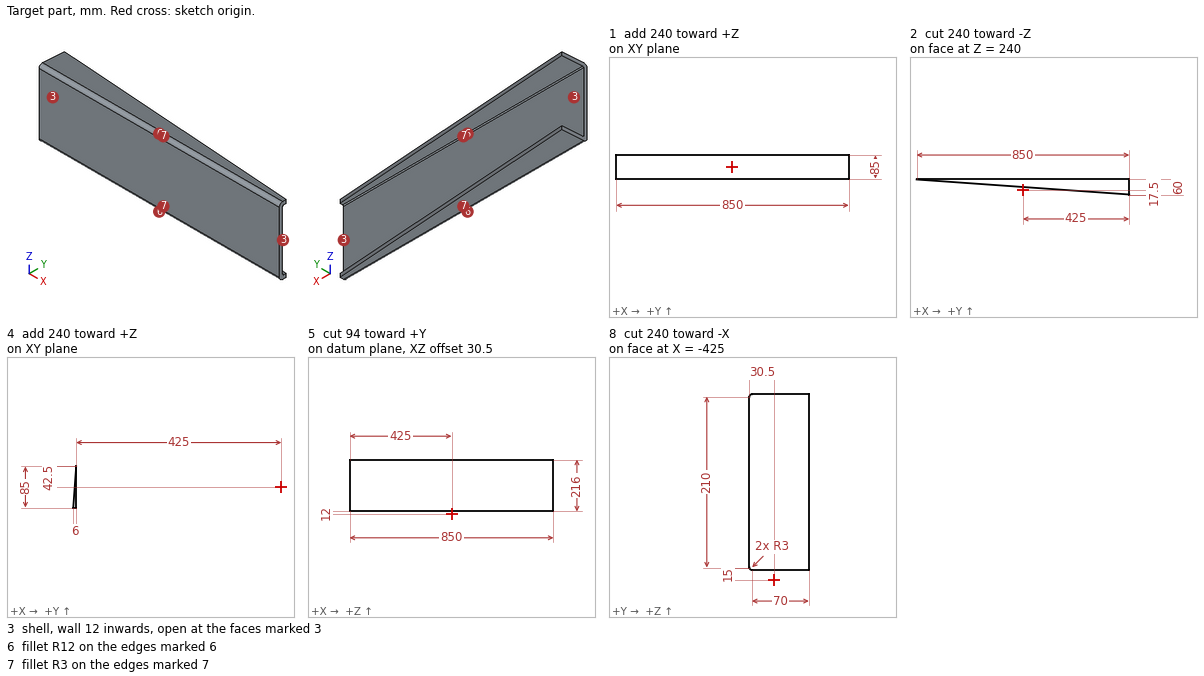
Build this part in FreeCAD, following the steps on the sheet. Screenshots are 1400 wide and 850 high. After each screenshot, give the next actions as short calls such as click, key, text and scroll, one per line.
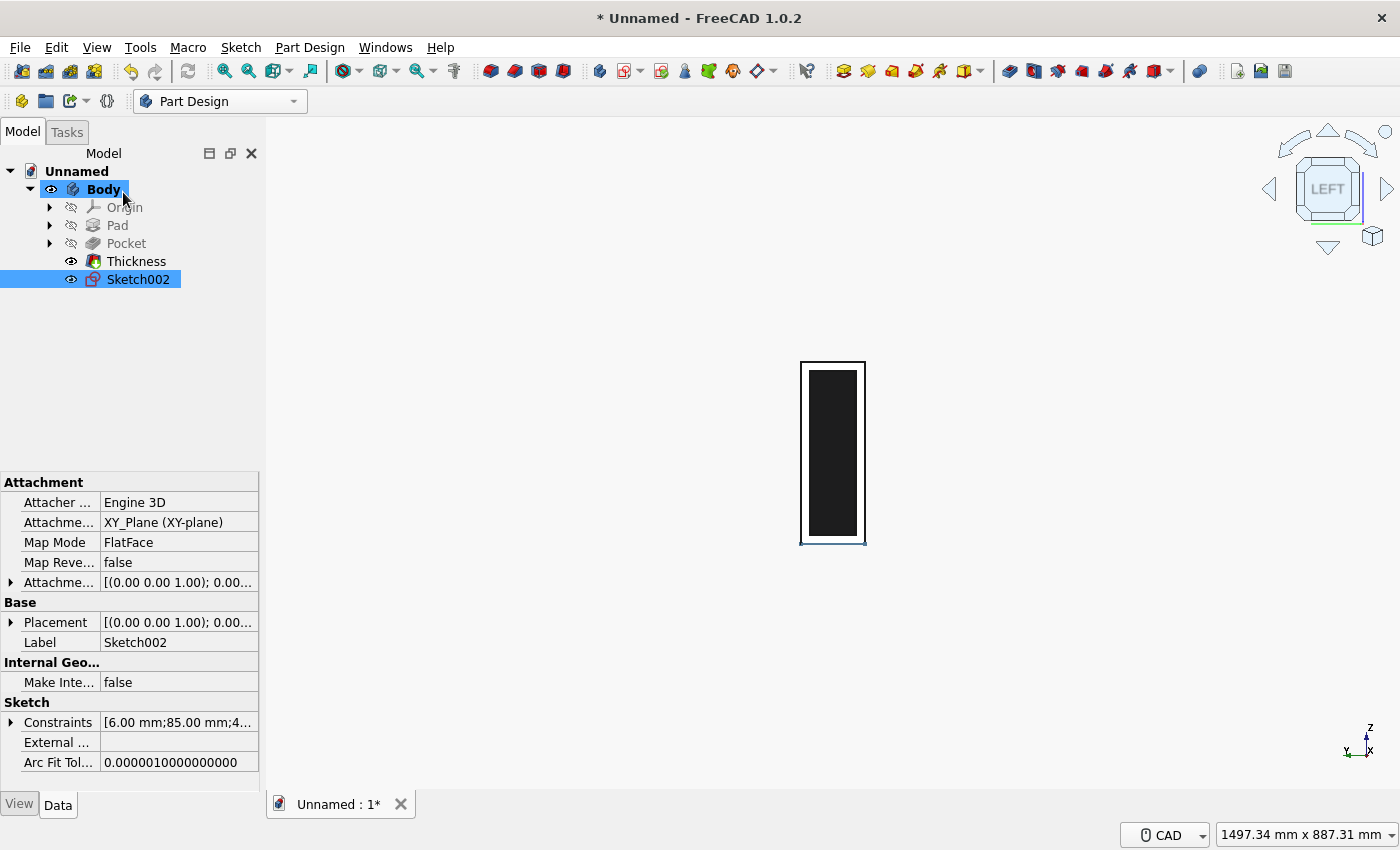
click(844, 72)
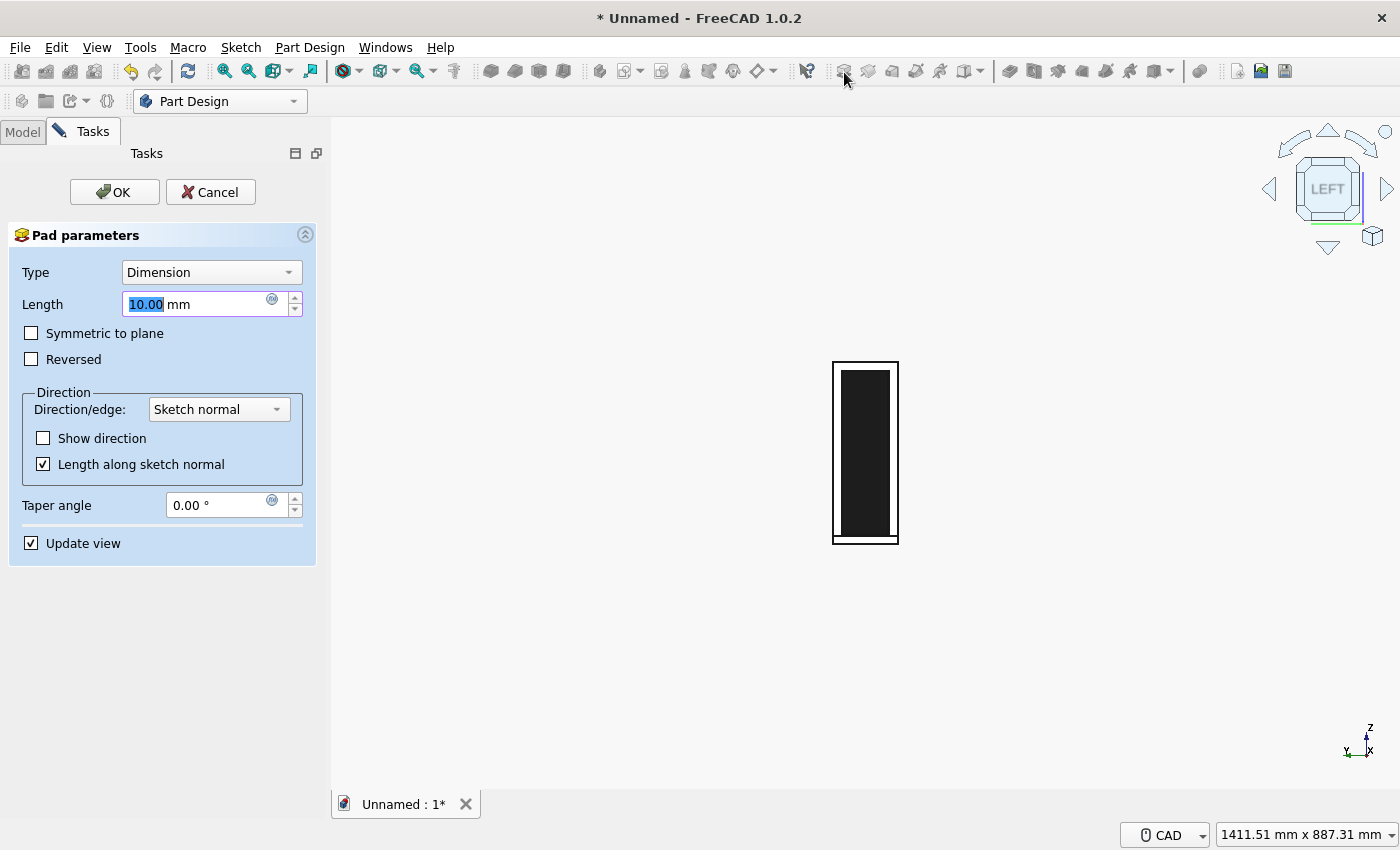
text(240)
key(Tab)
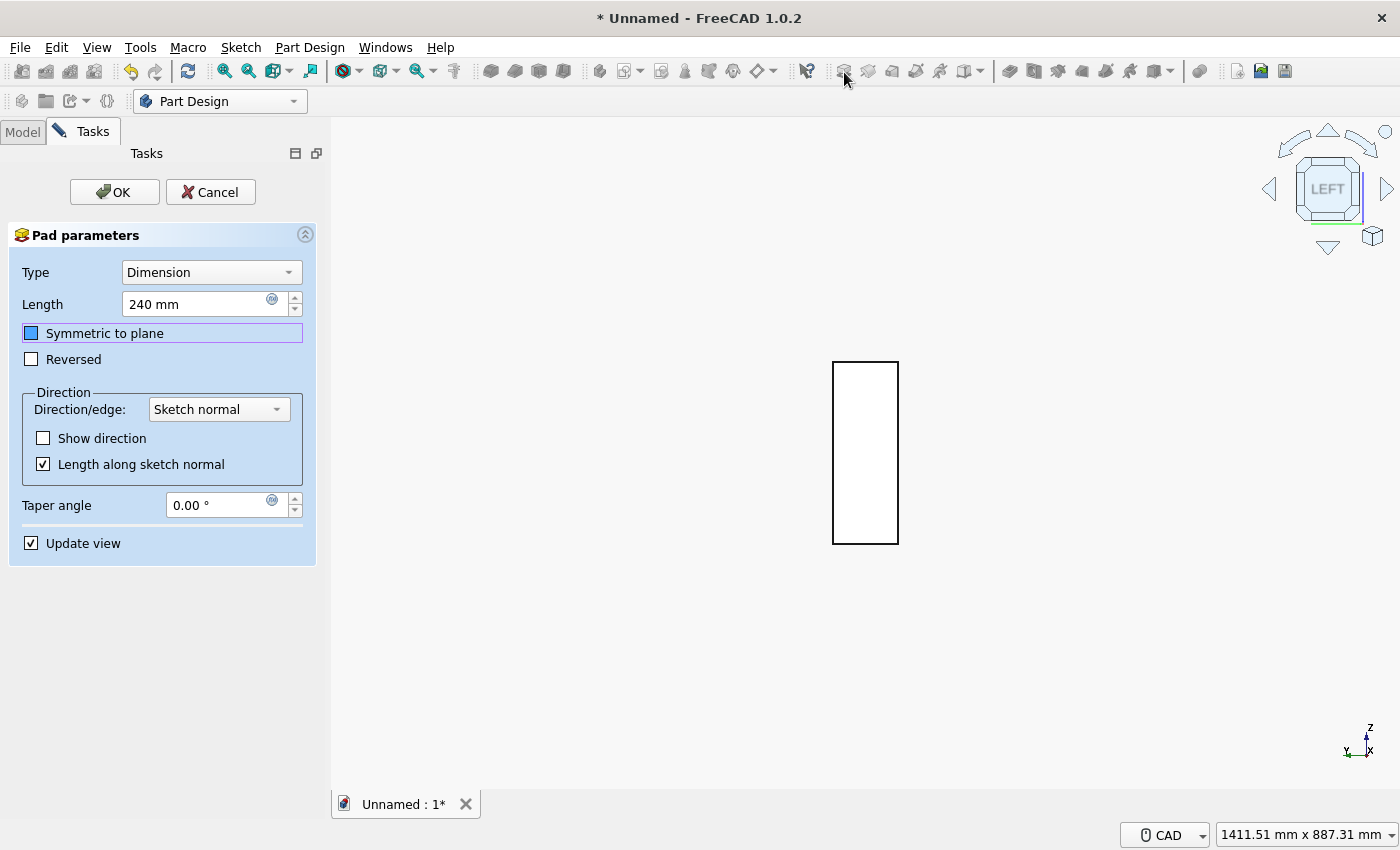
click(115, 192)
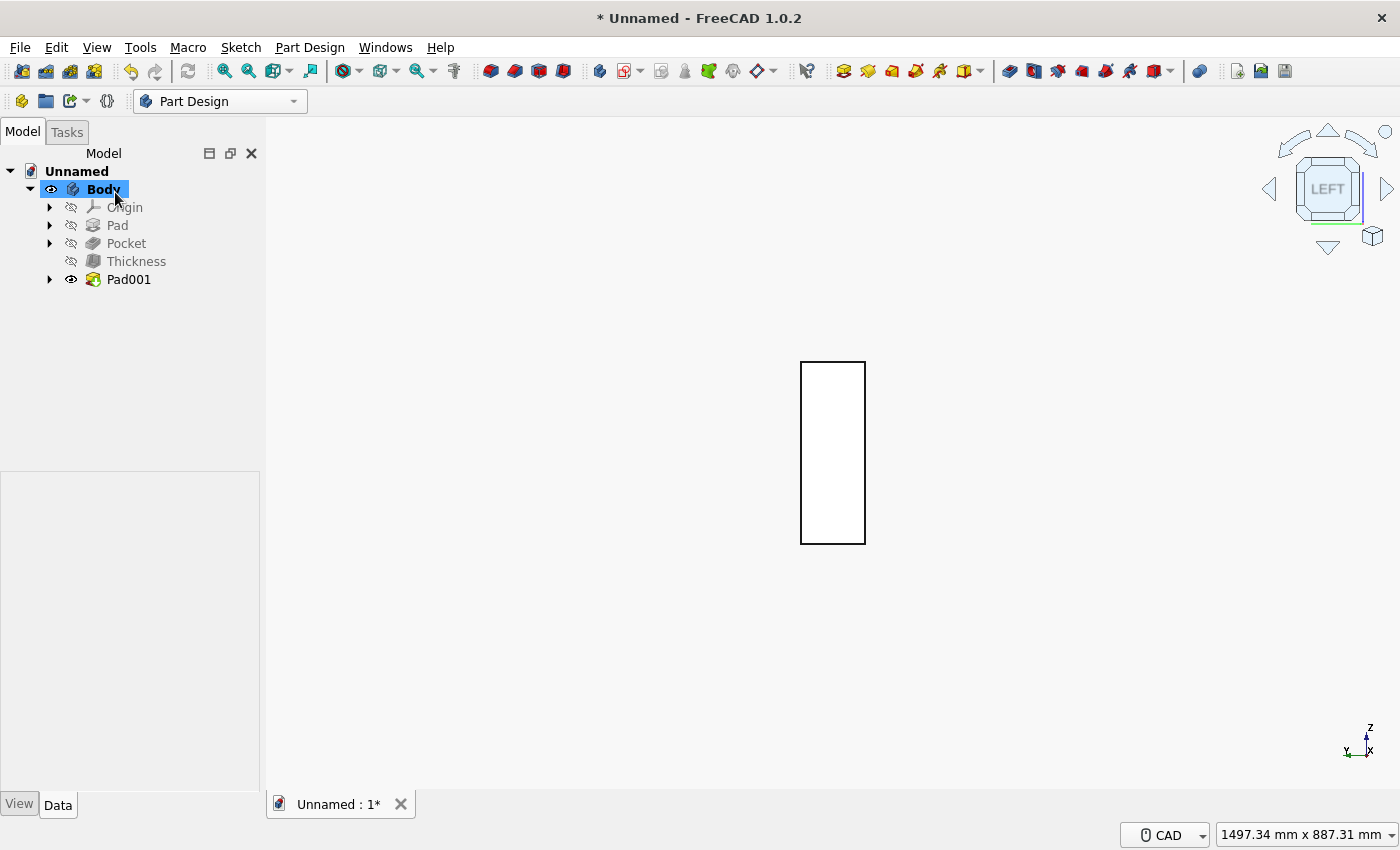
key(v)
key(f)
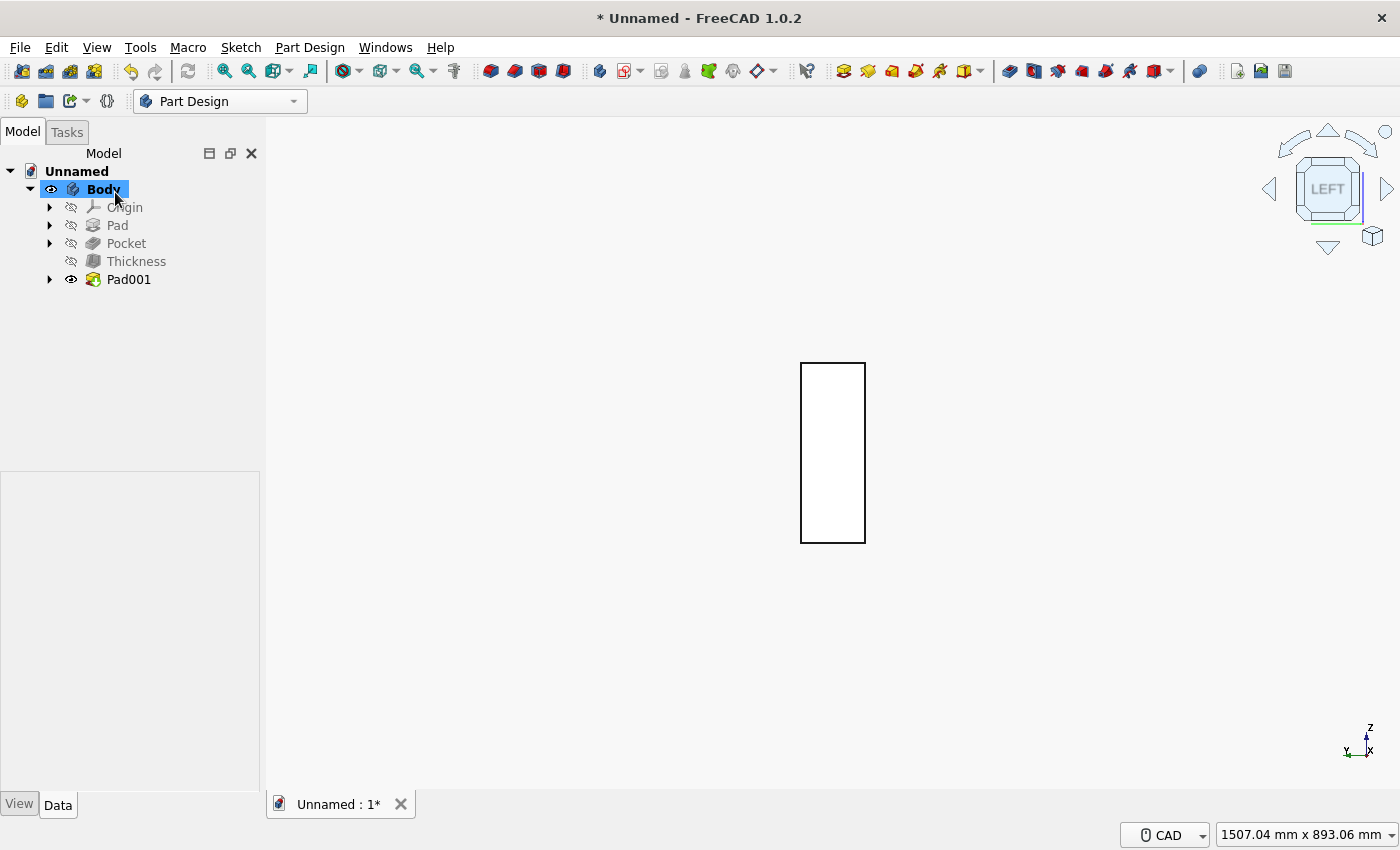
click(50, 207)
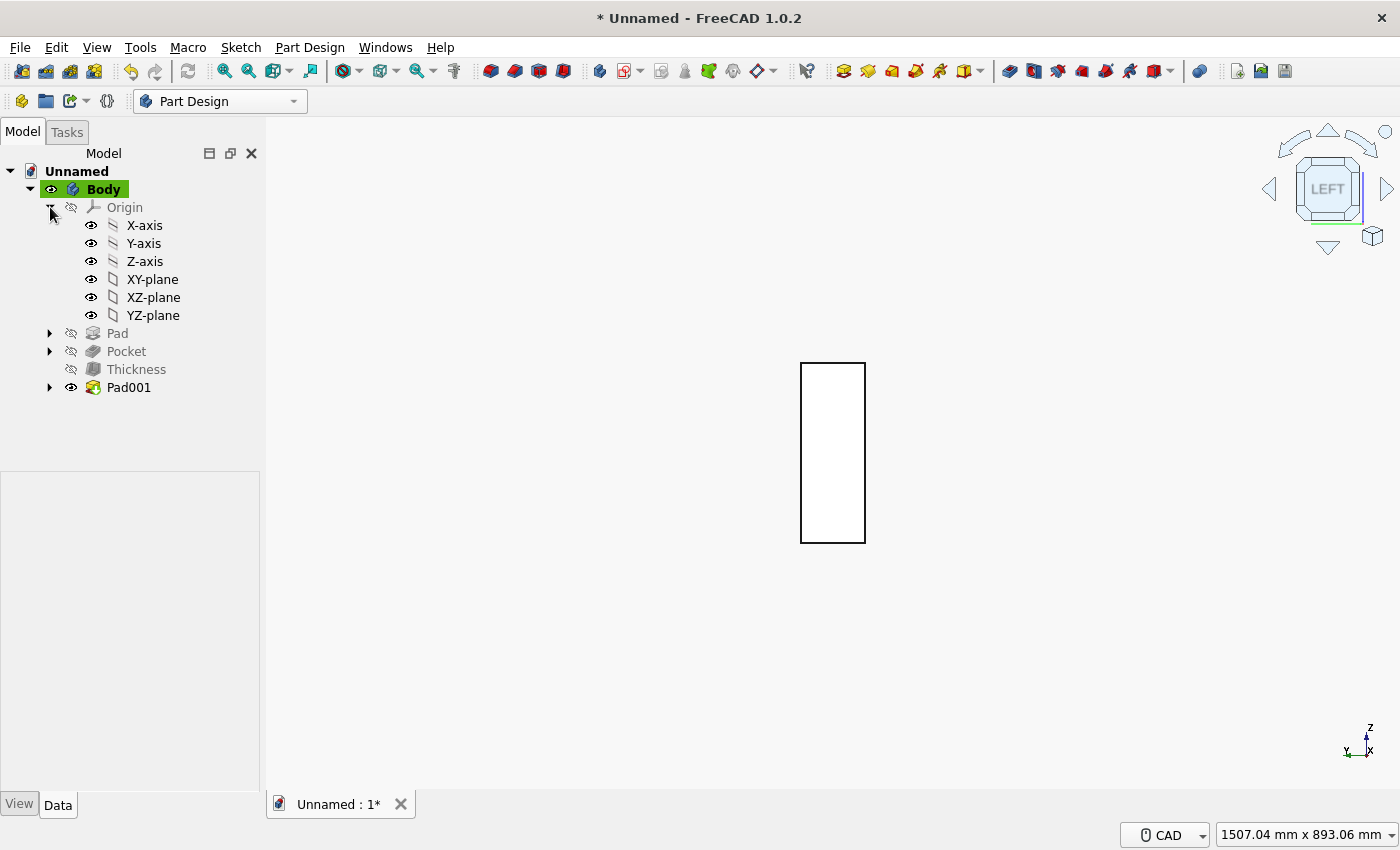
click(136, 297)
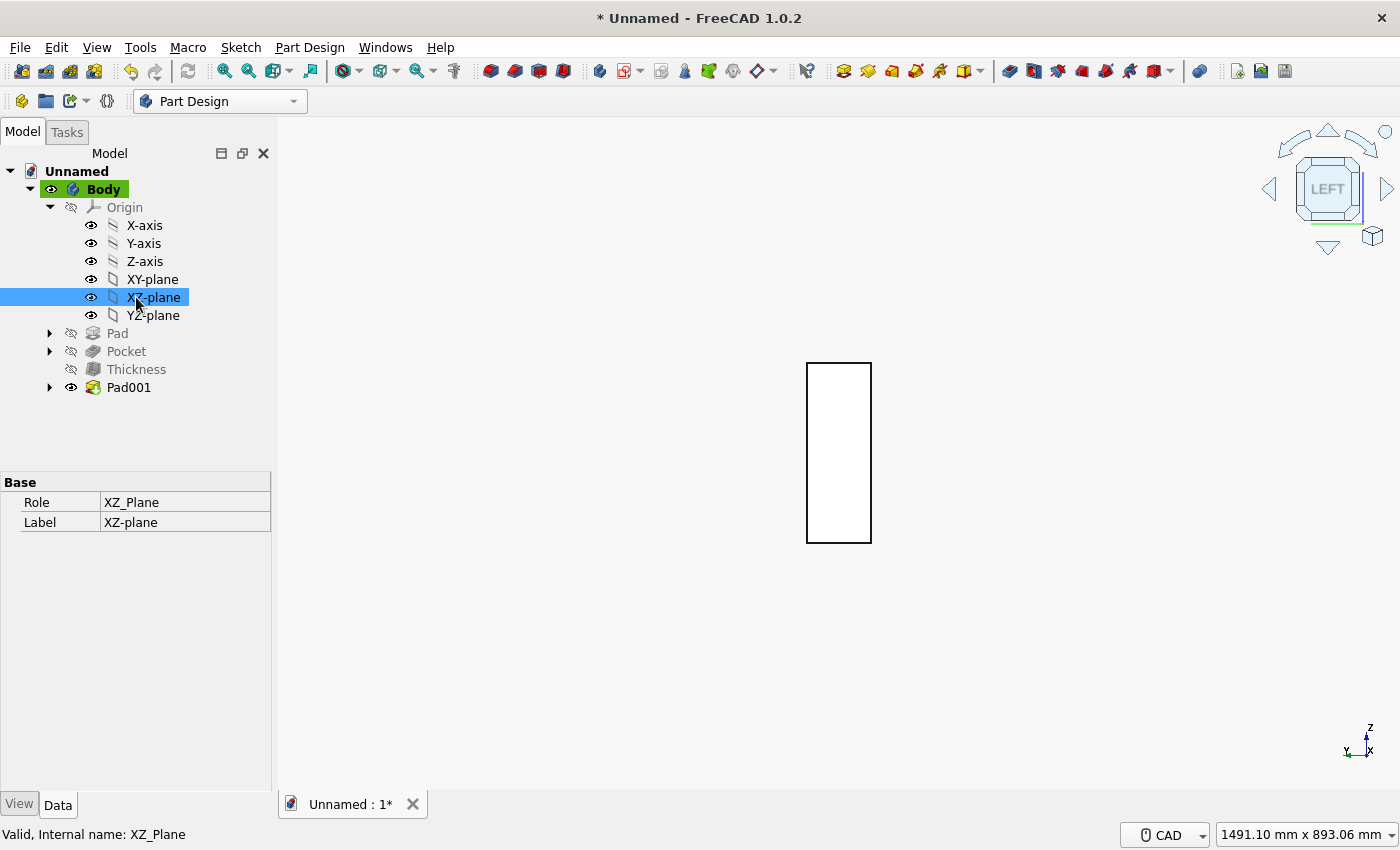
click(758, 72)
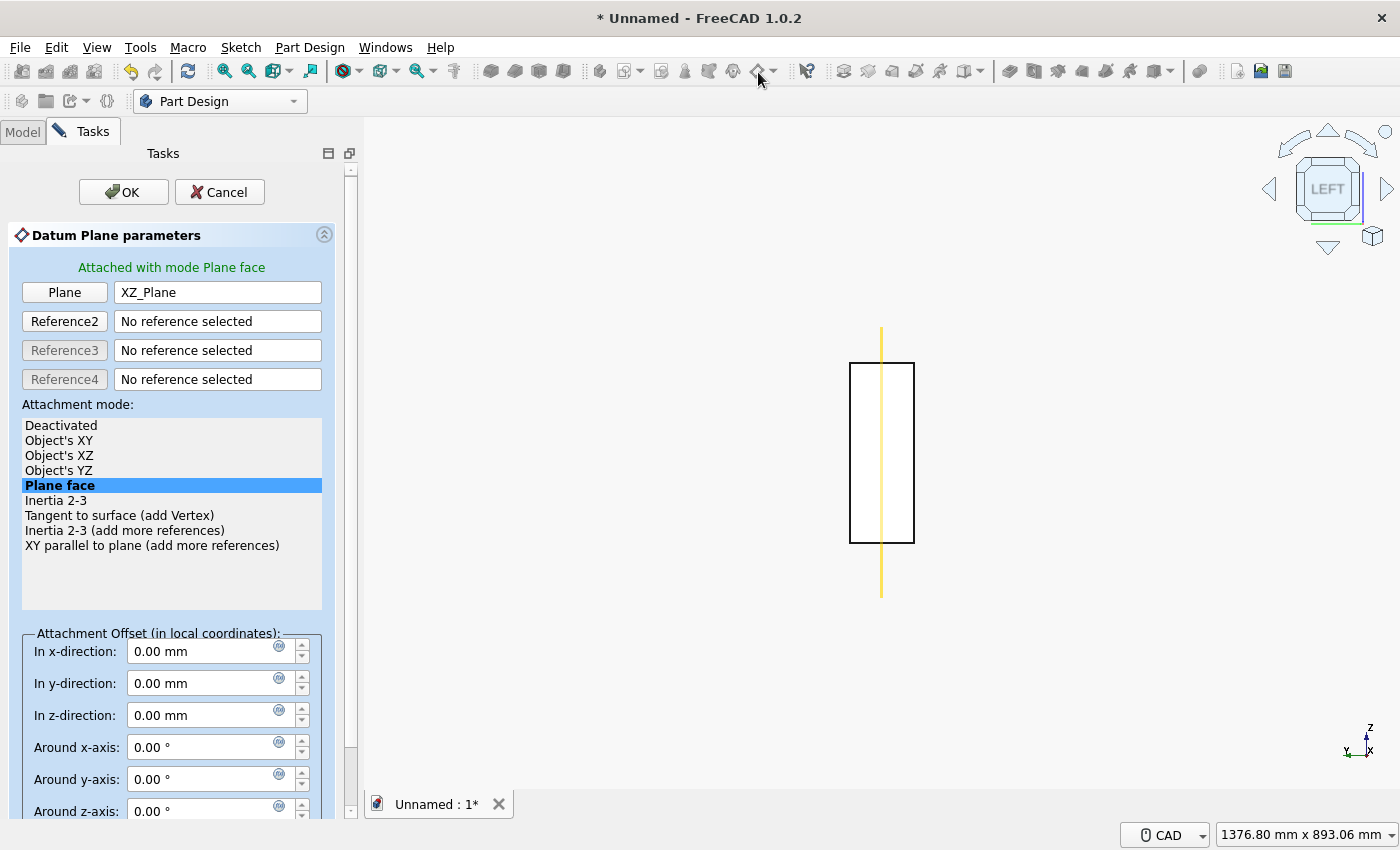
triple_click(210, 715)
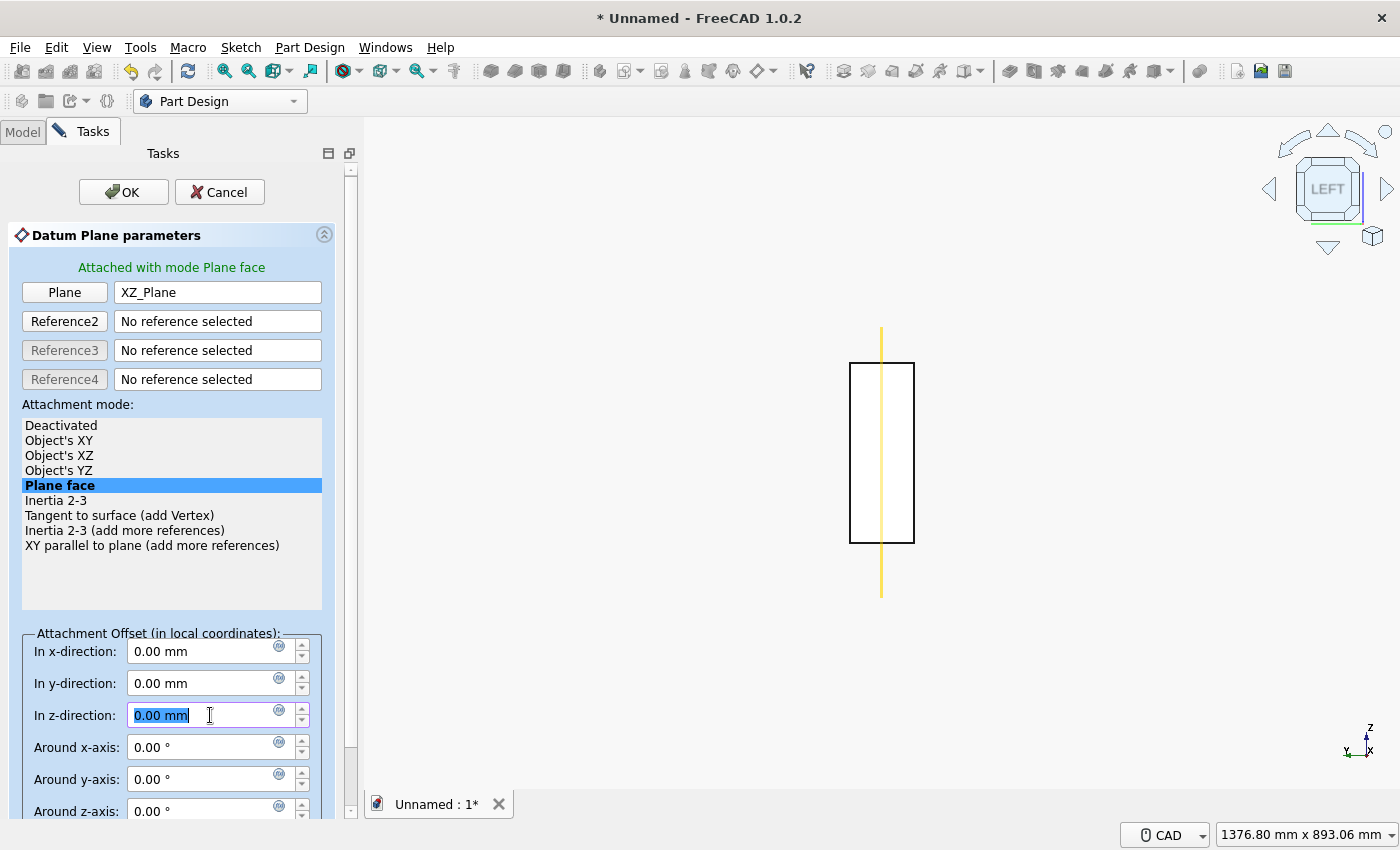
text(30.5)
key(Tab)